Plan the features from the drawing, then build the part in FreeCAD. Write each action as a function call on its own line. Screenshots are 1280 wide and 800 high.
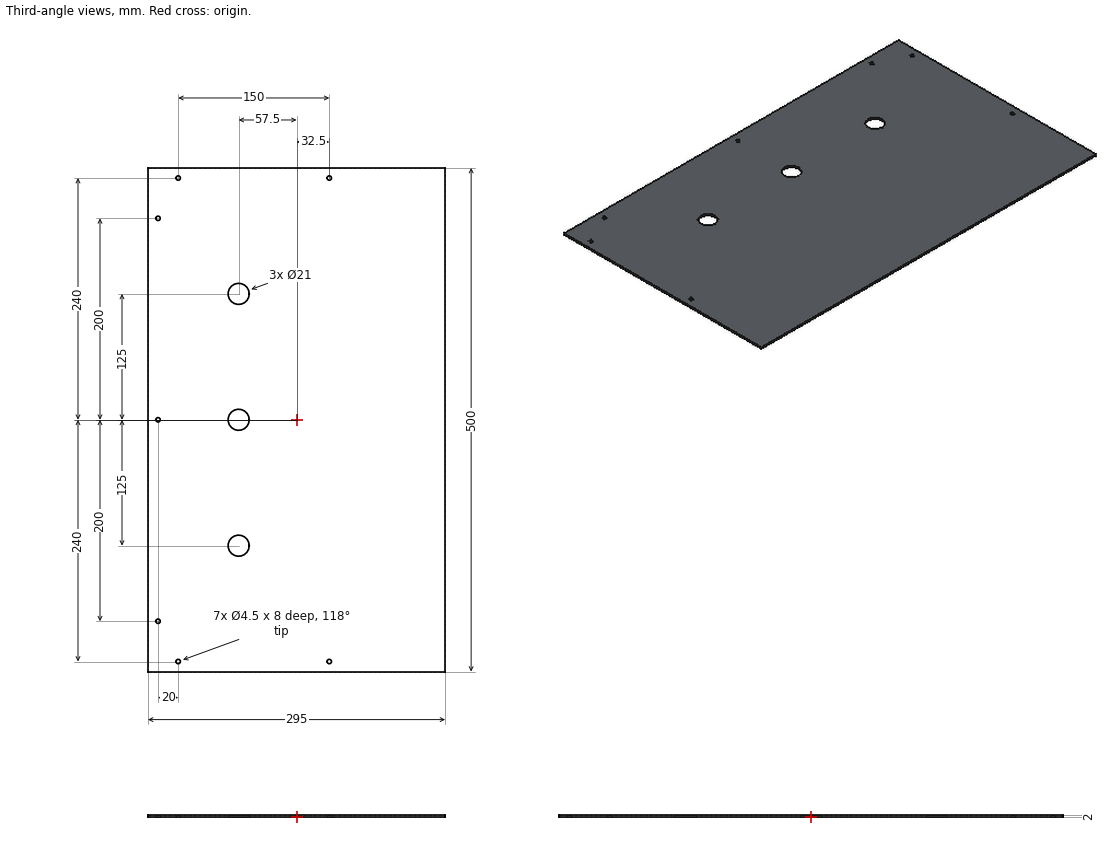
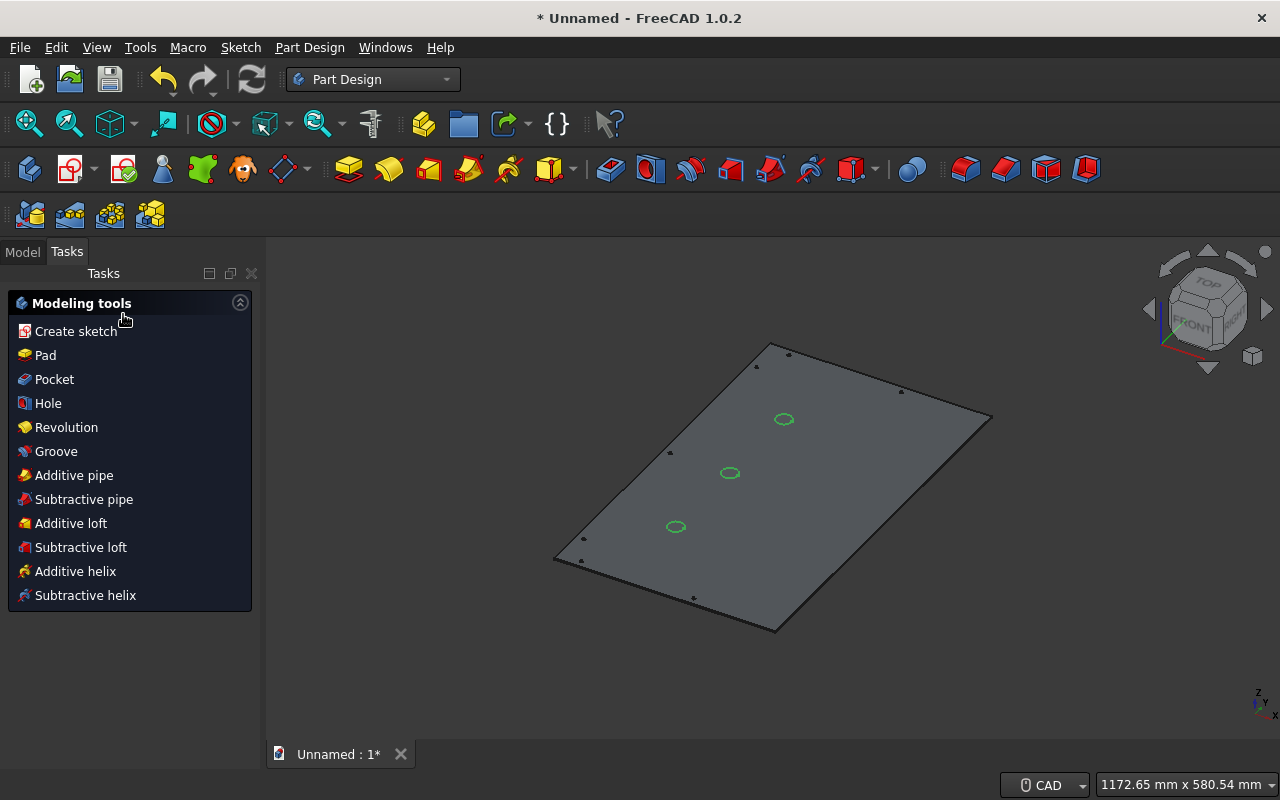
click(612, 170)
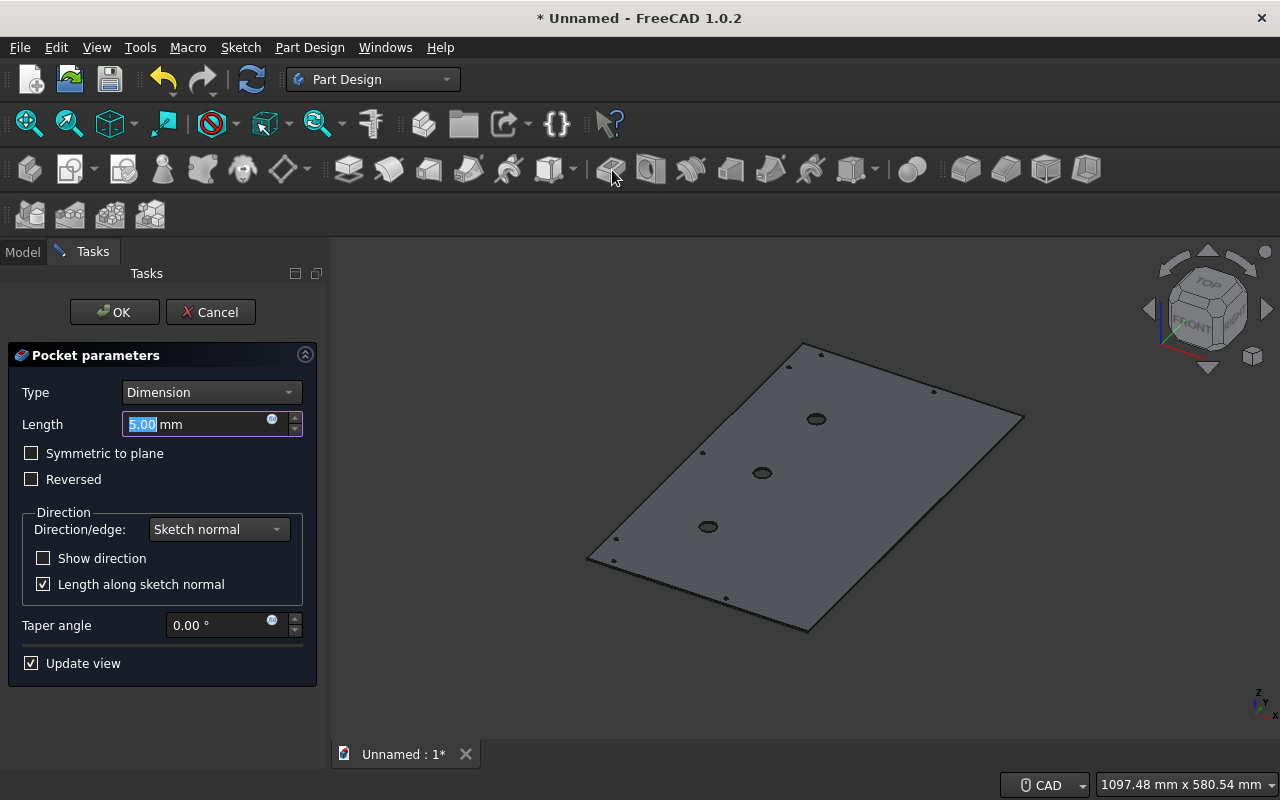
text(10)
key(Tab)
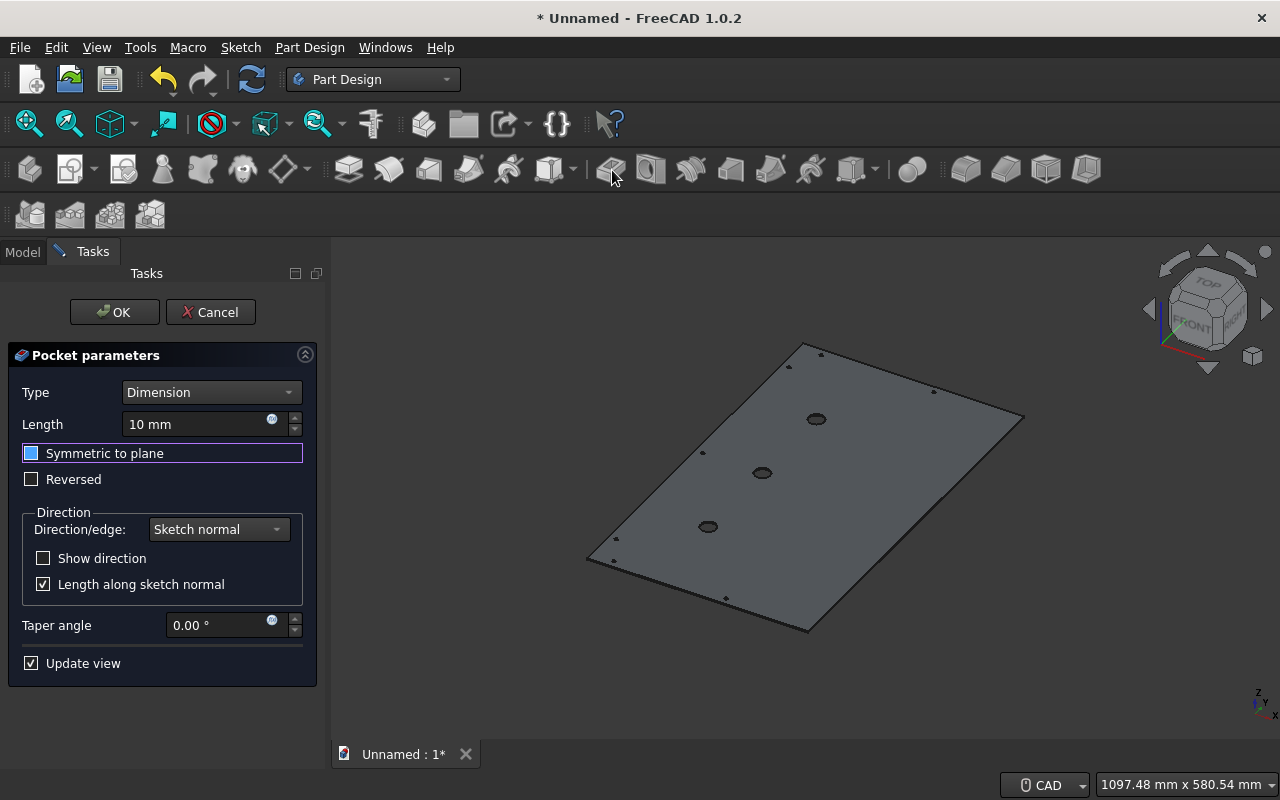
click(115, 312)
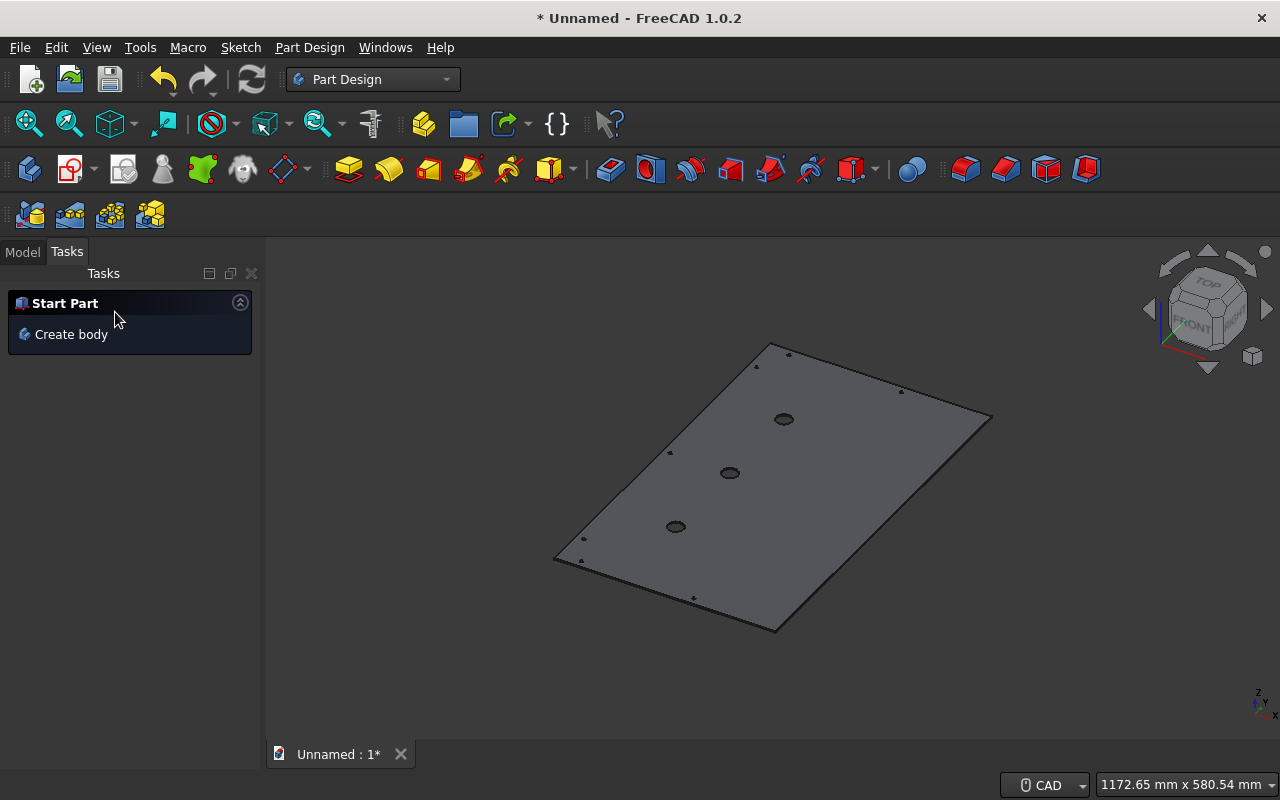
key(0)